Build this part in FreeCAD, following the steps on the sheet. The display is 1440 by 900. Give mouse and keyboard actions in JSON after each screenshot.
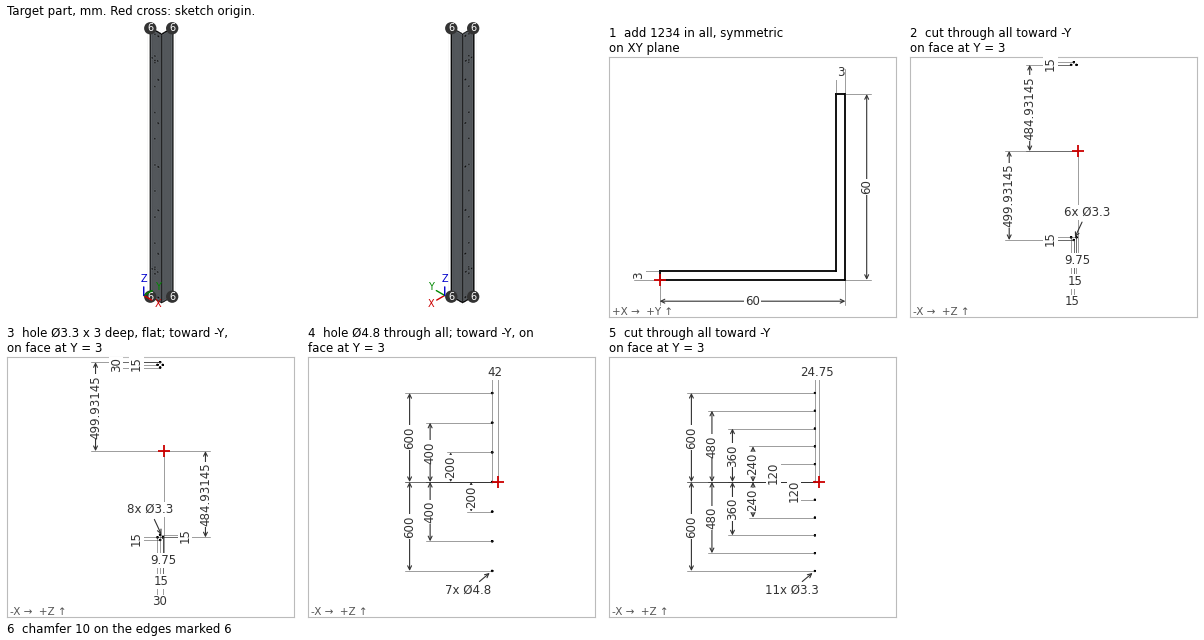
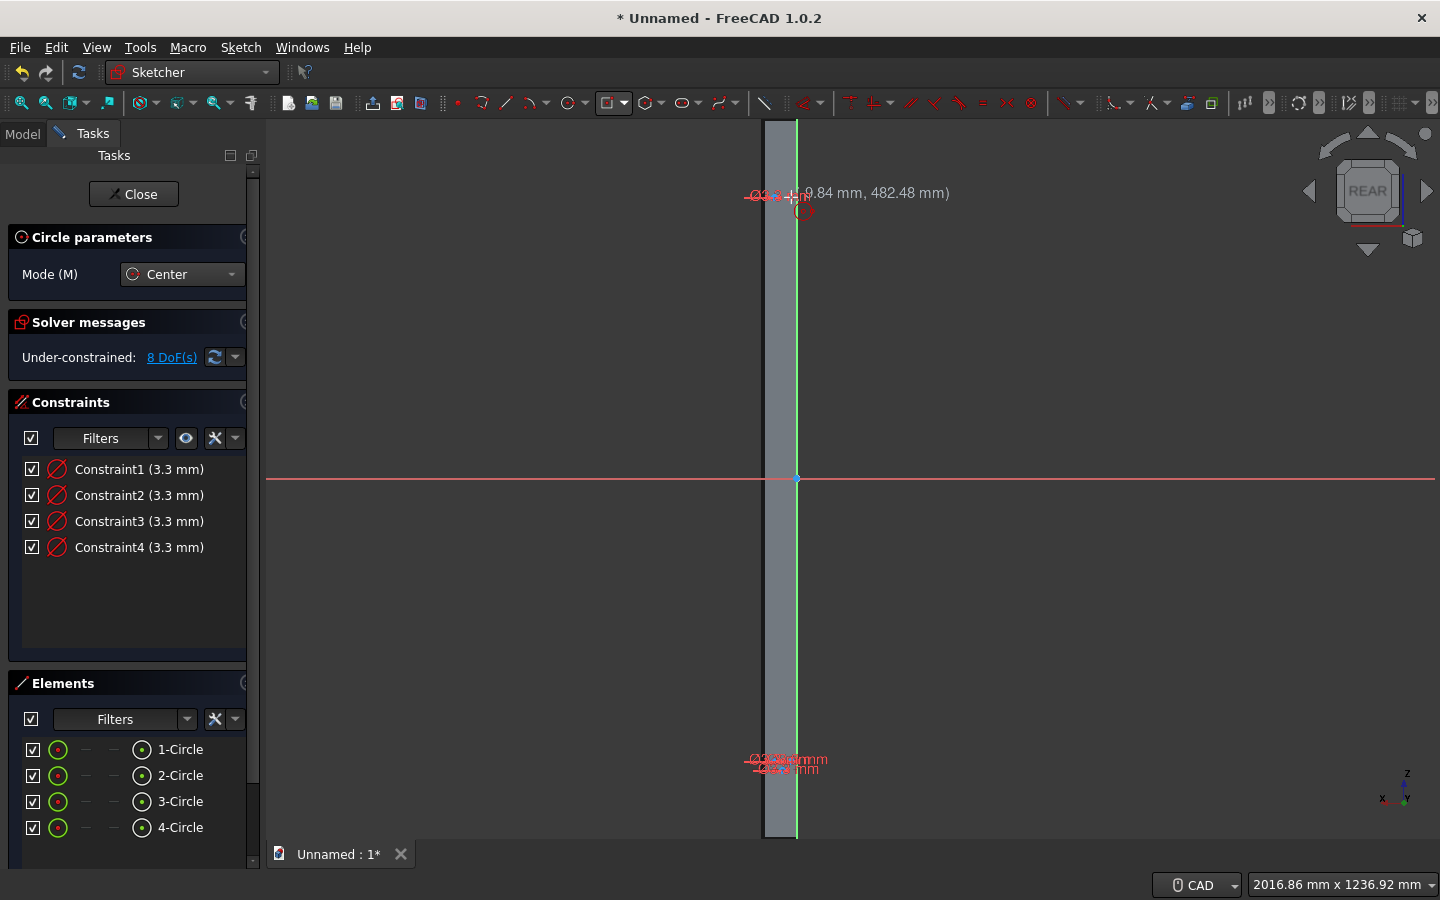
{"action": "scroll", "coordinate": [791, 197], "scroll_direction": "up", "scroll_amount": 6}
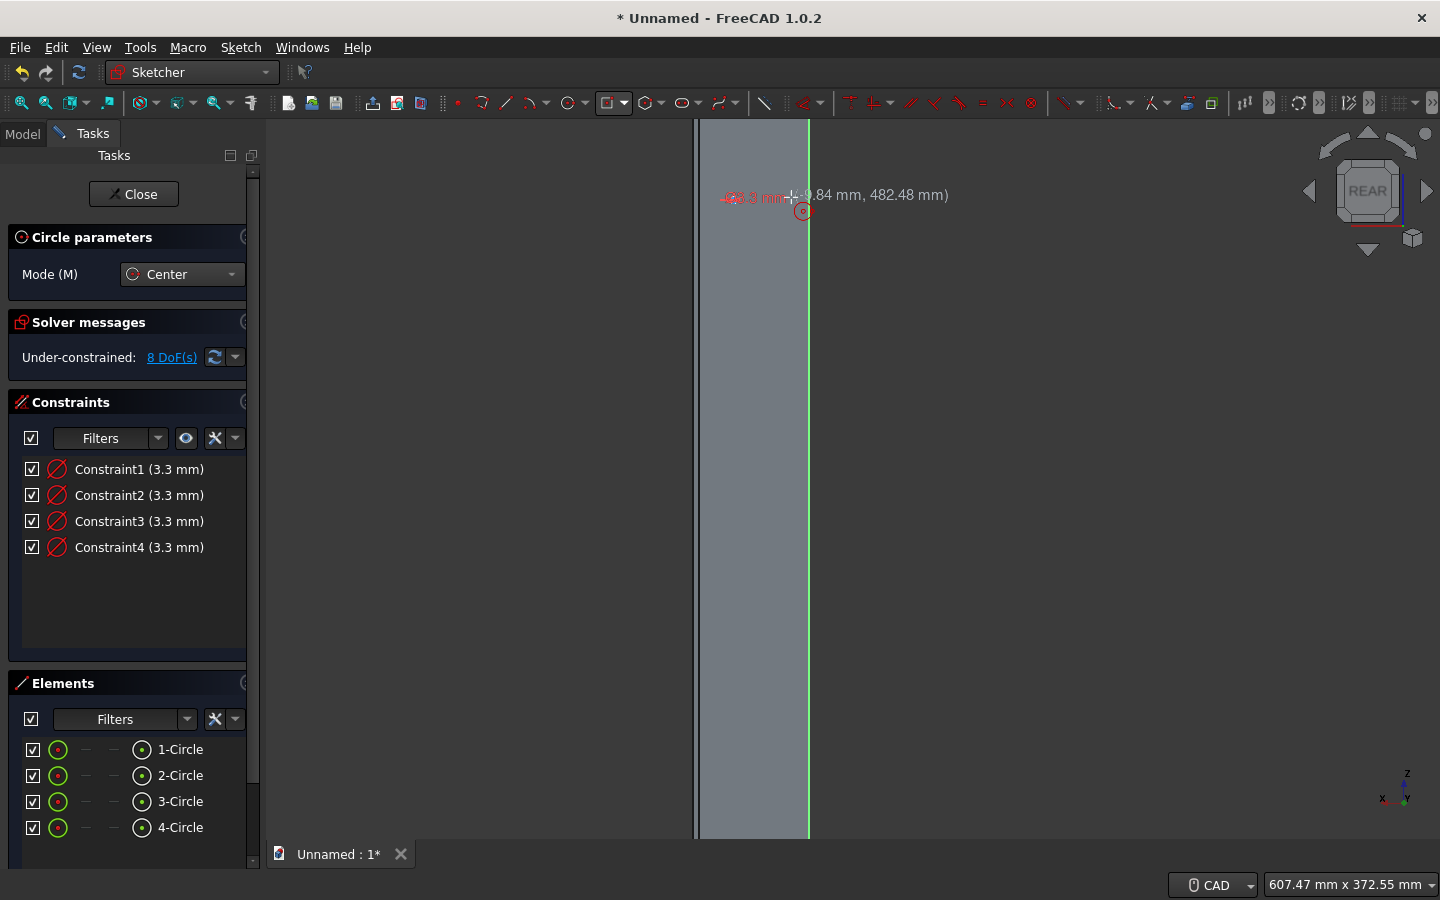
{"action": "left_click", "coordinate": [790, 195]}
{"action": "mouse_move", "coordinate": [792, 193]}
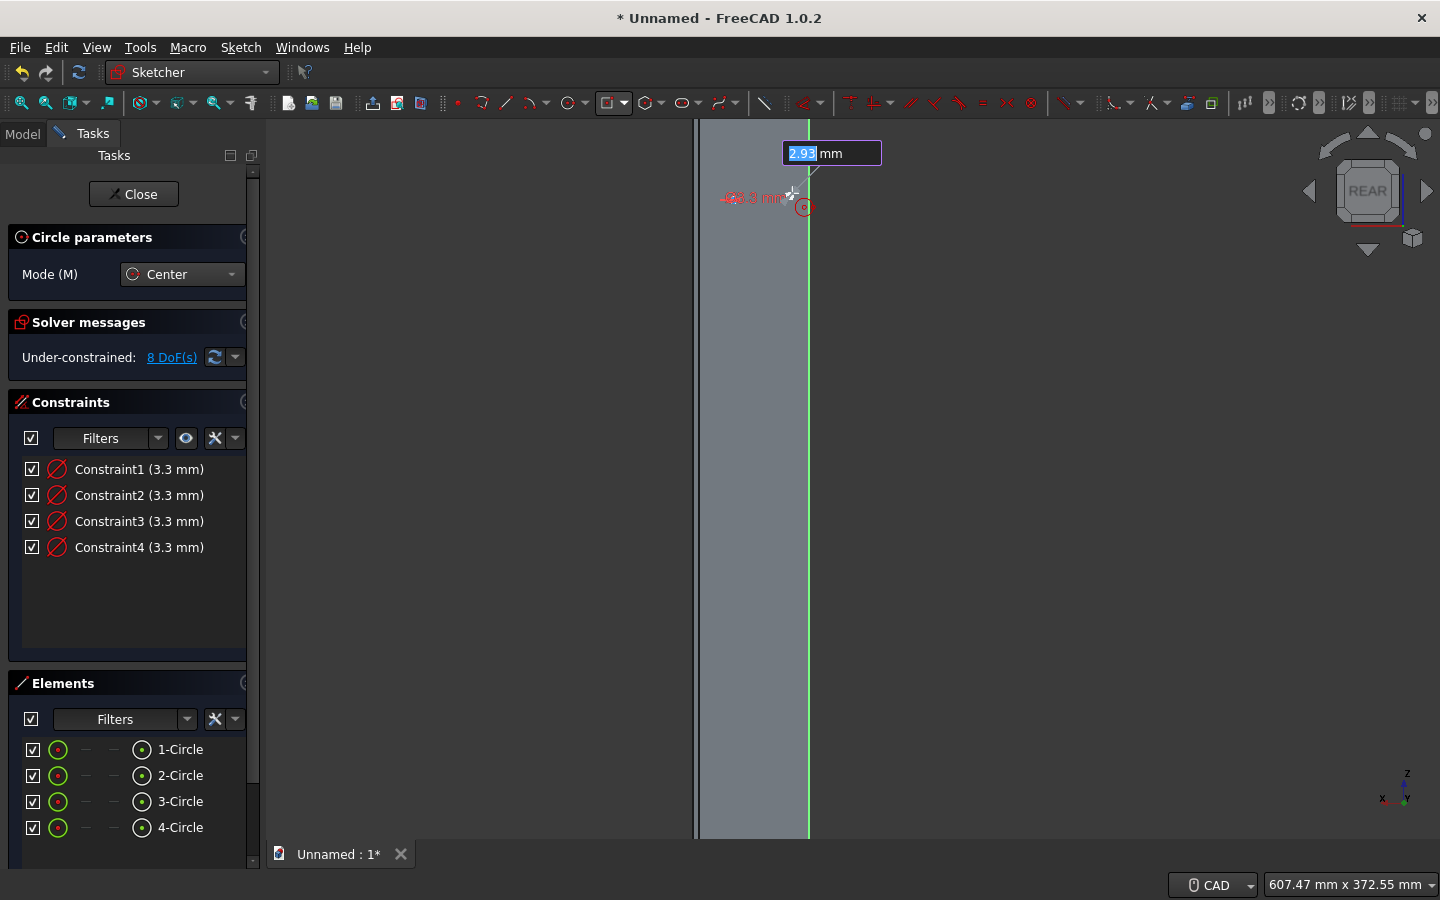
{"action": "type", "text": "3.3"}
{"action": "key", "text": "Return"}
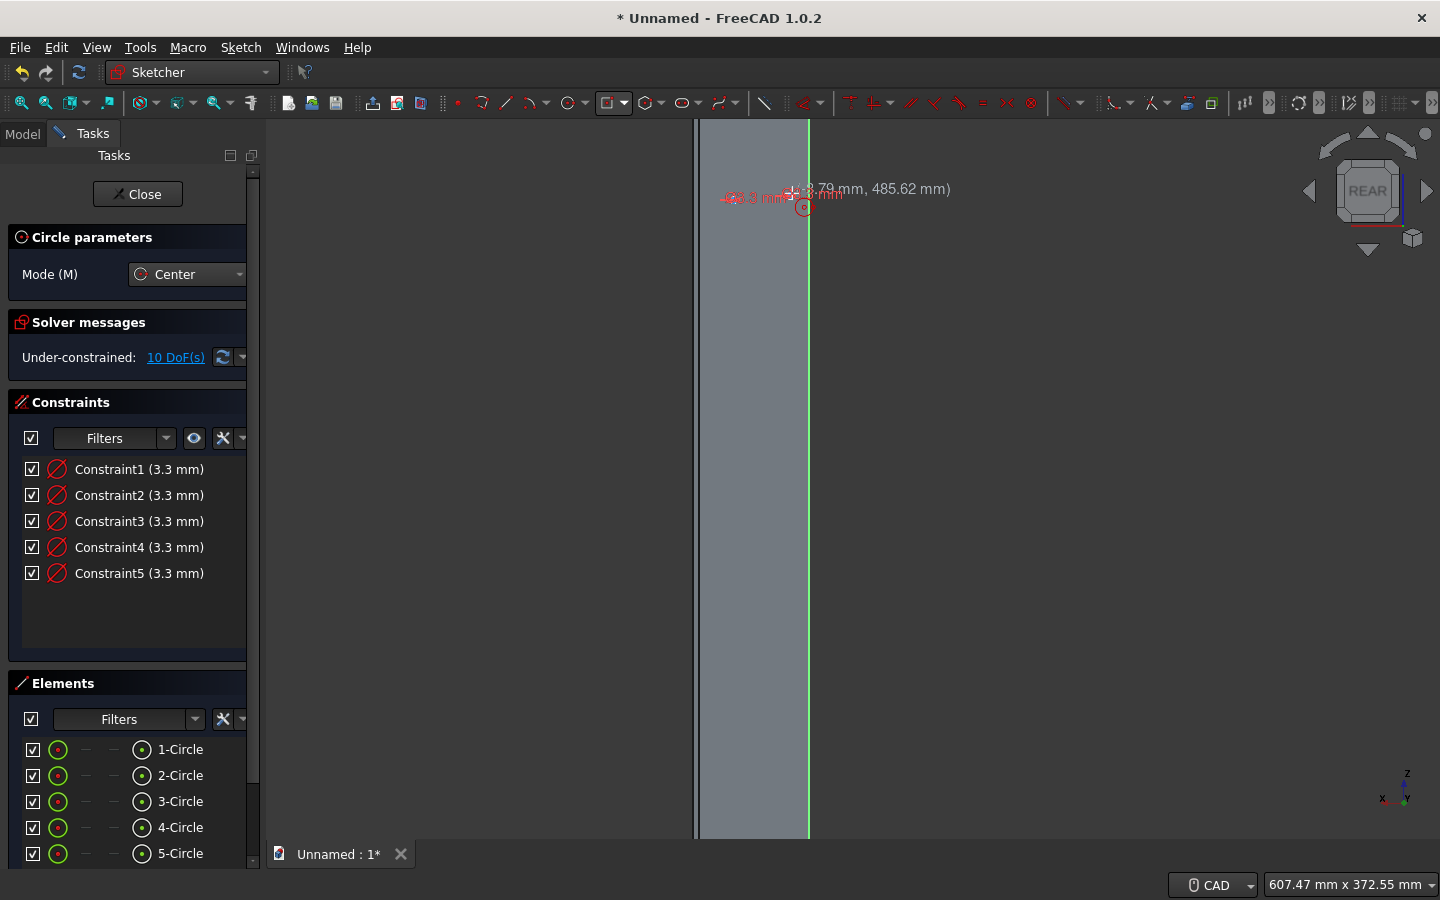
{"action": "scroll", "coordinate": [761, 166], "scroll_direction": "up", "scroll_amount": 10}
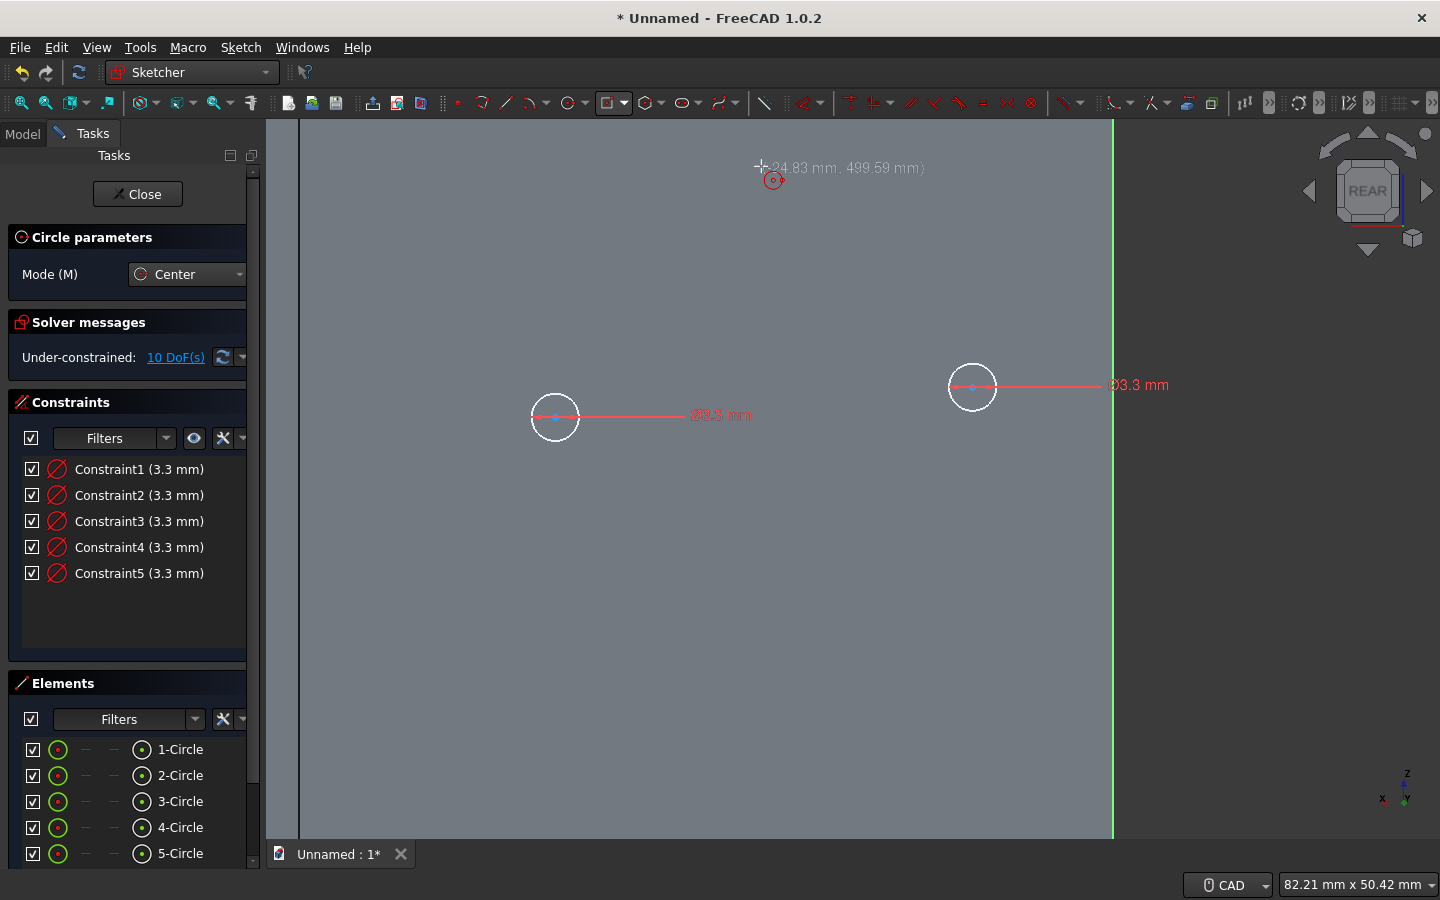
{"action": "scroll", "coordinate": [783, 189], "scroll_direction": "down", "scroll_amount": 16}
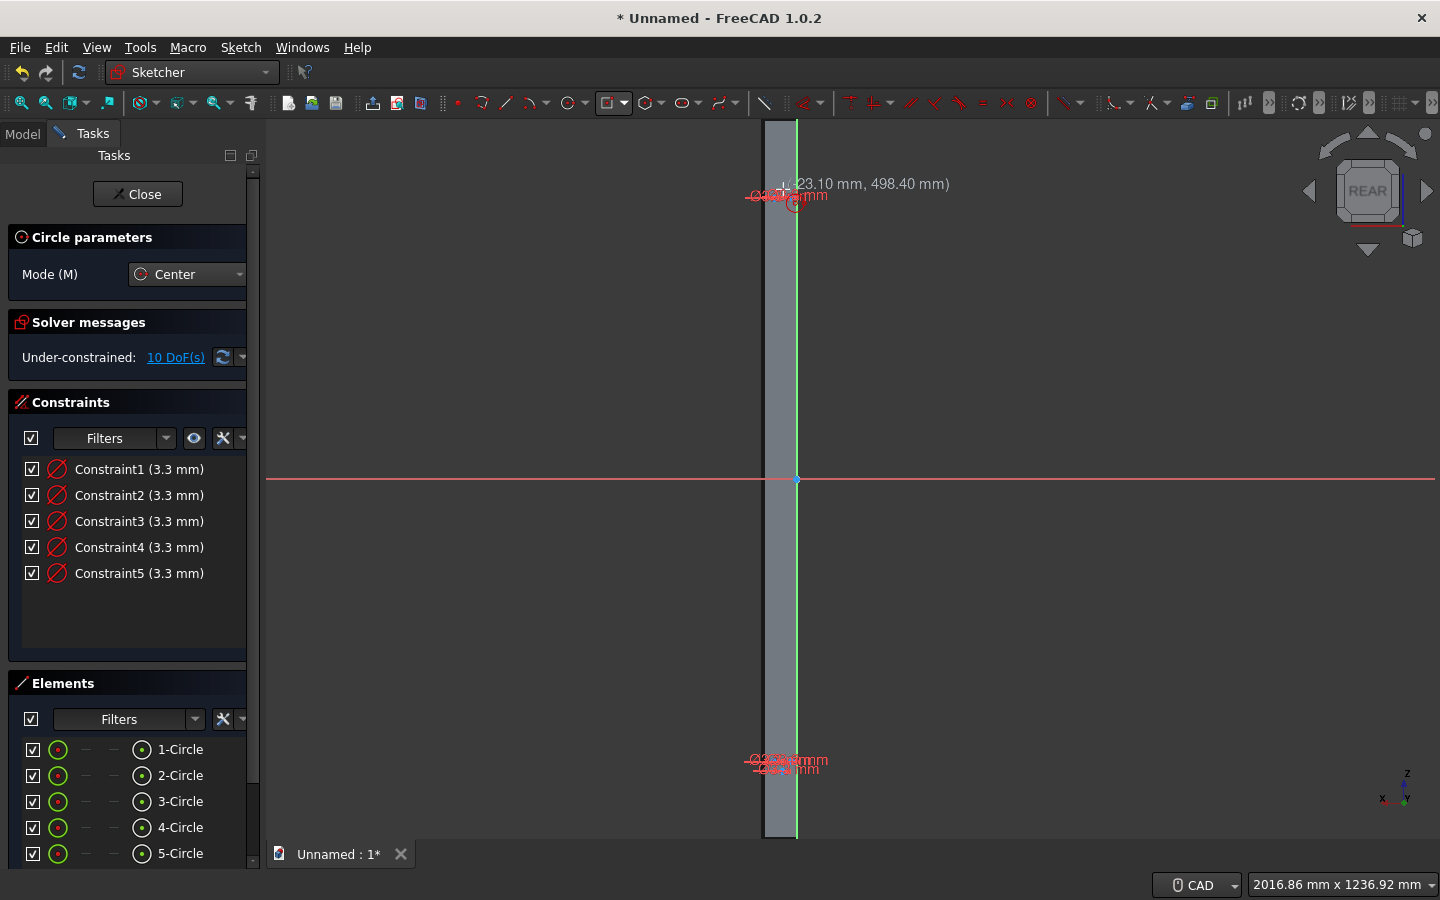
{"action": "scroll", "coordinate": [782, 188], "scroll_direction": "up", "scroll_amount": 2}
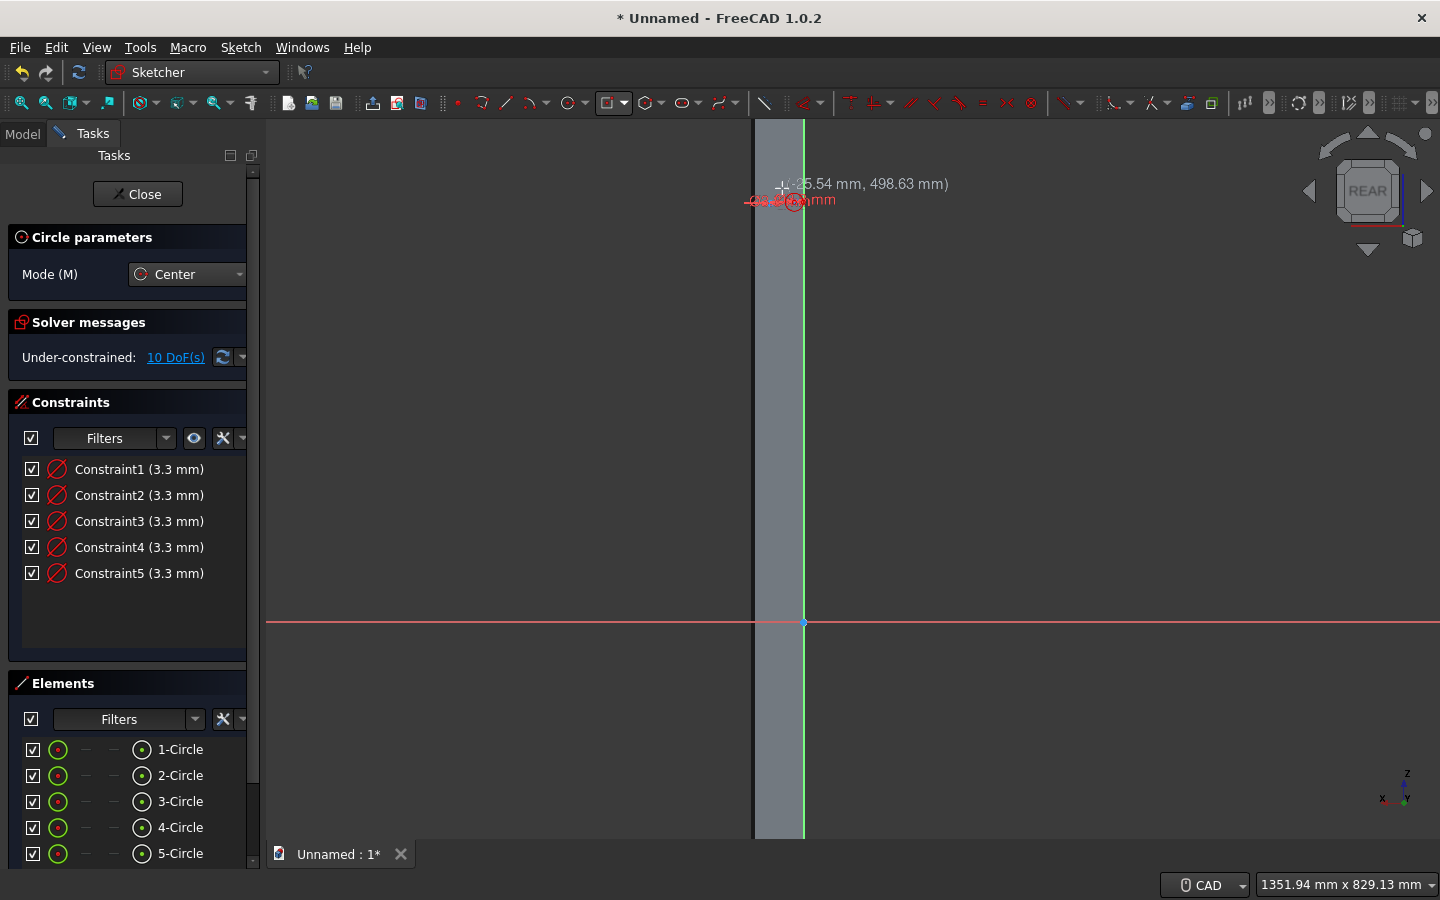
{"action": "left_click", "coordinate": [782, 188]}
{"action": "mouse_move", "coordinate": [783, 187]}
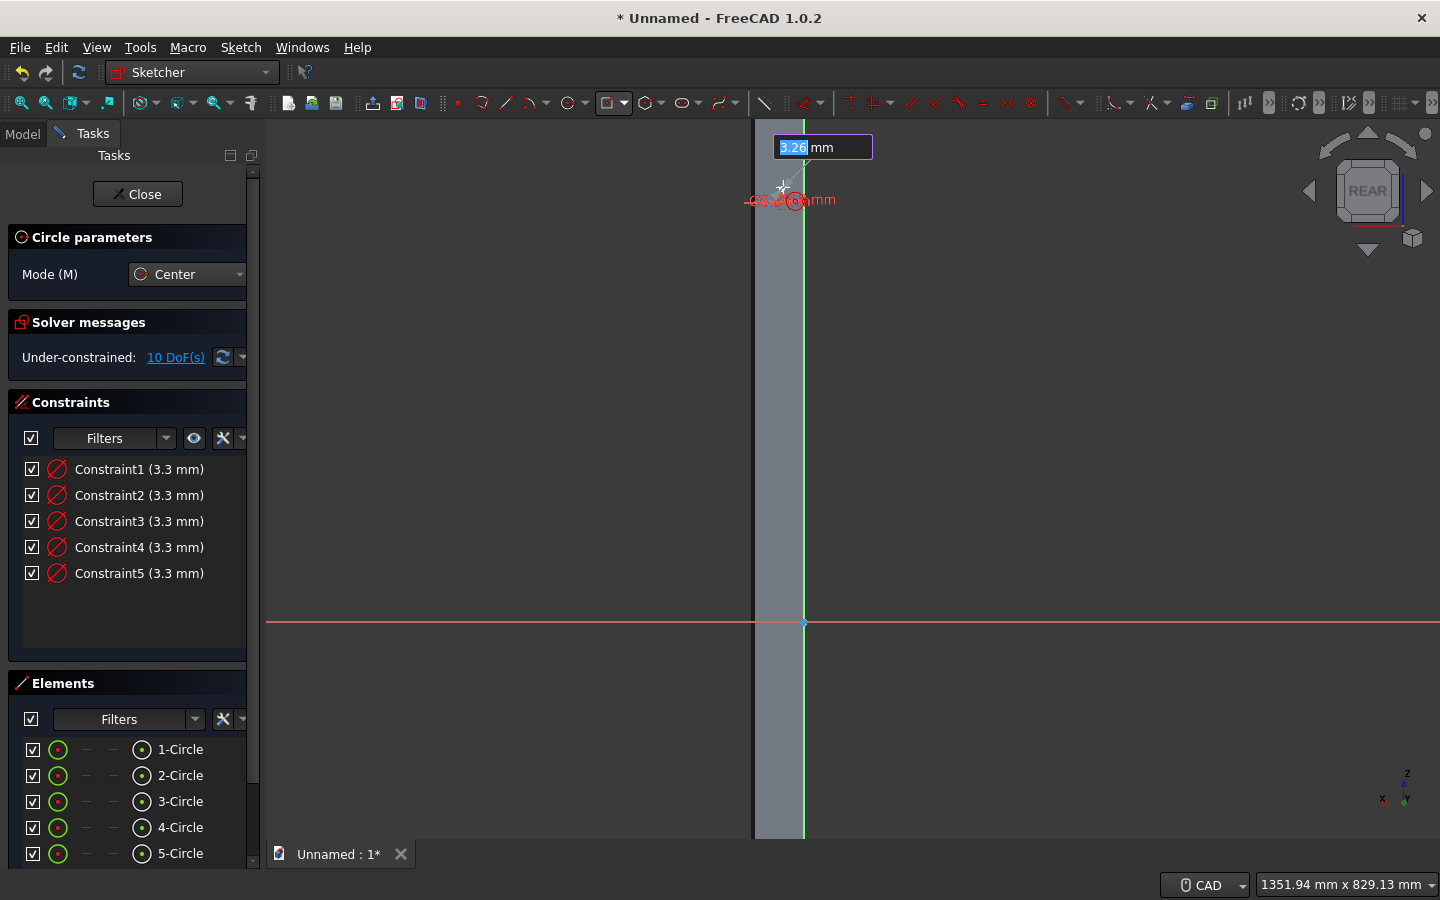
{"action": "type", "text": "3.3"}
{"action": "key", "text": "Return"}
{"action": "key", "text": "Escape"}